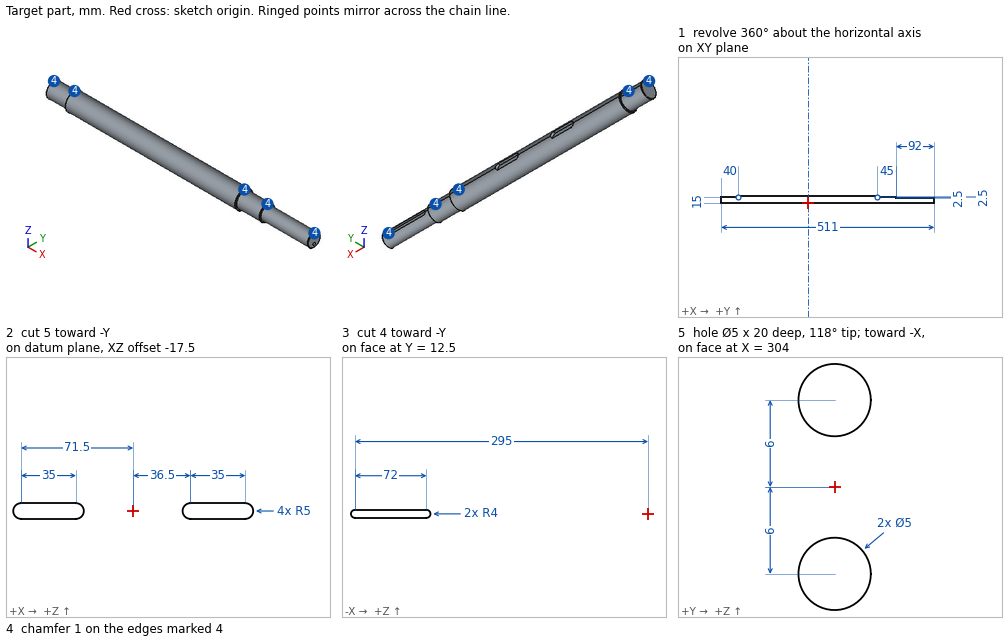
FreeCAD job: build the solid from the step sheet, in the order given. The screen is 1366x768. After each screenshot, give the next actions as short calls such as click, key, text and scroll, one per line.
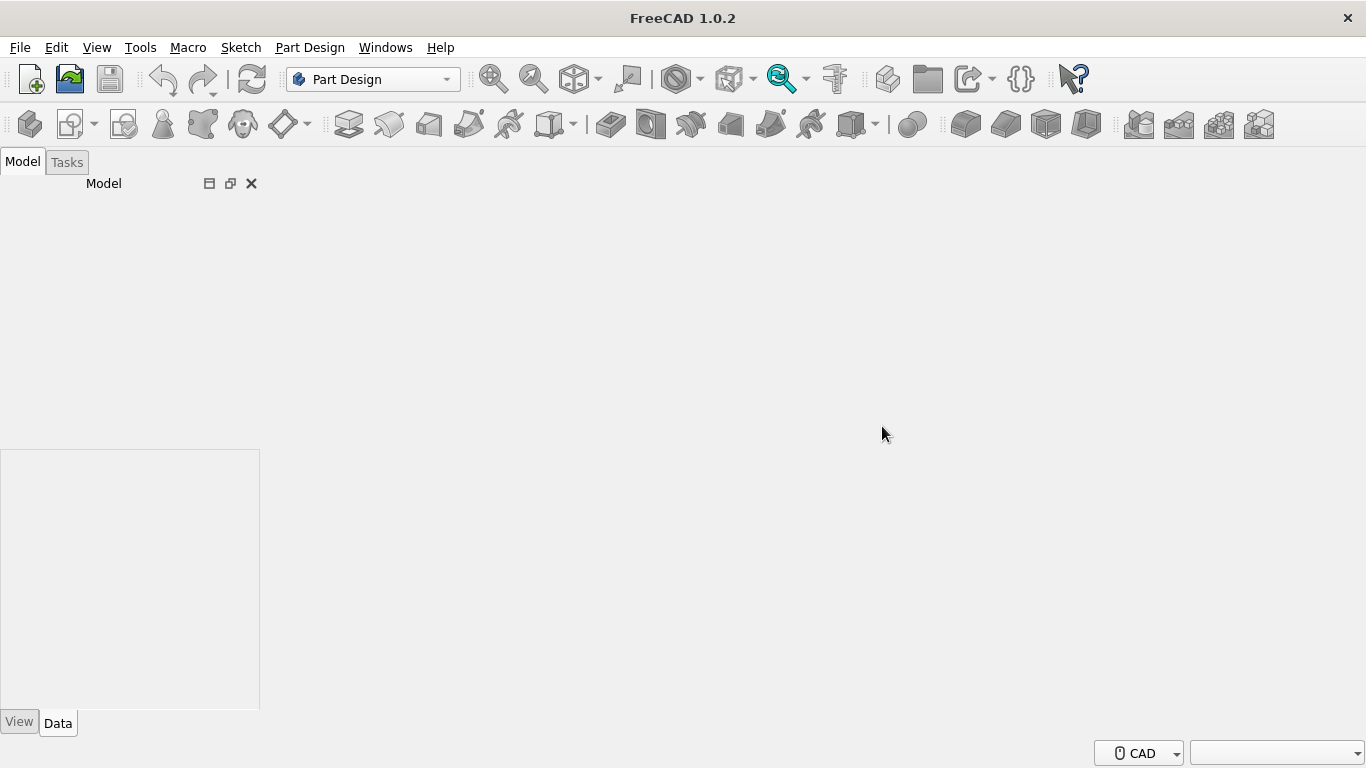
click(30, 80)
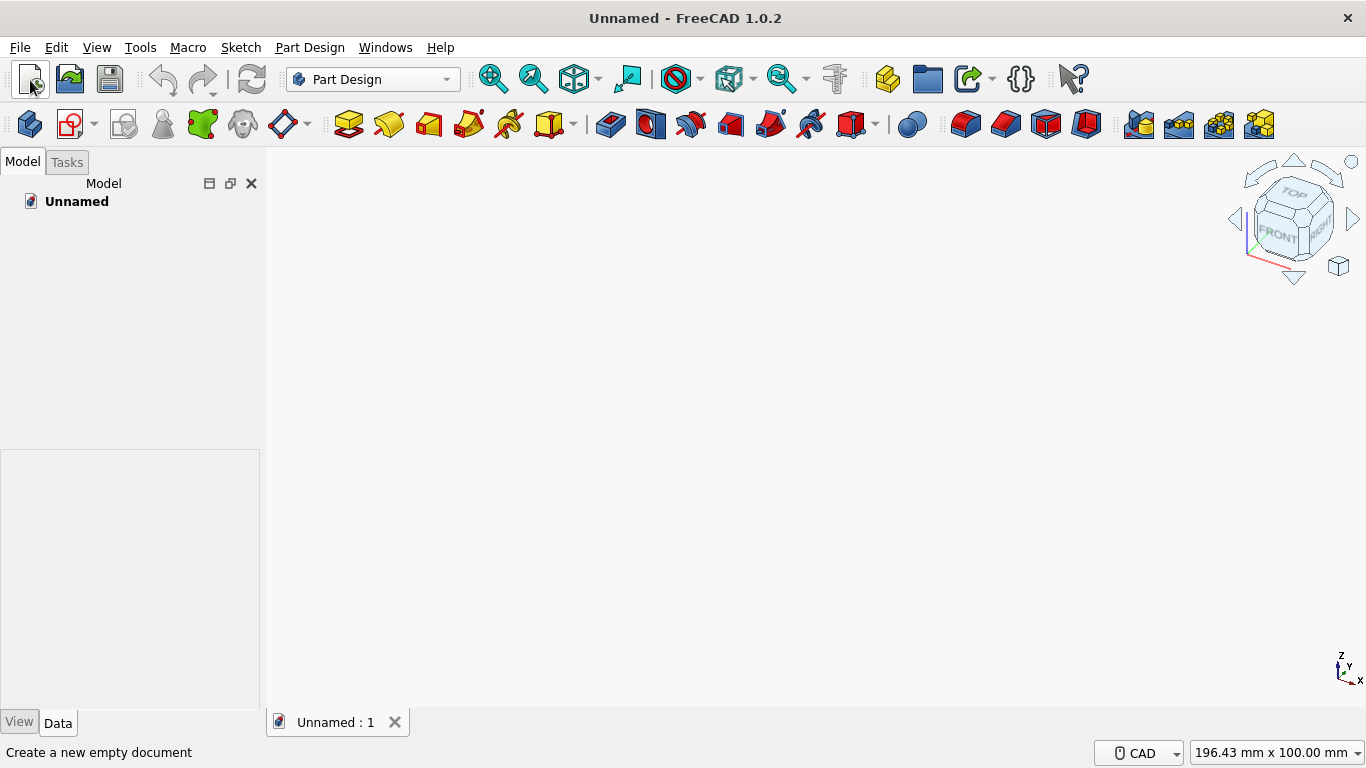
click(70, 124)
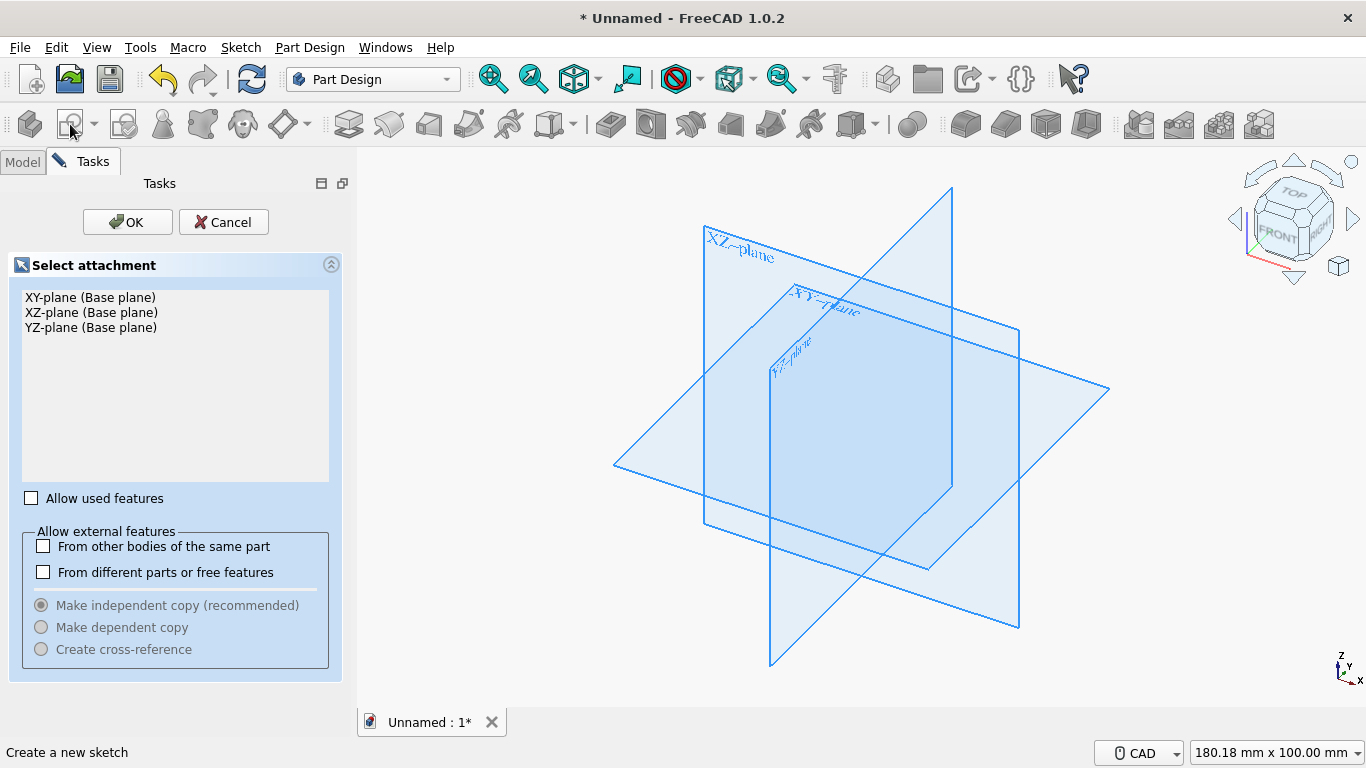
click(82, 298)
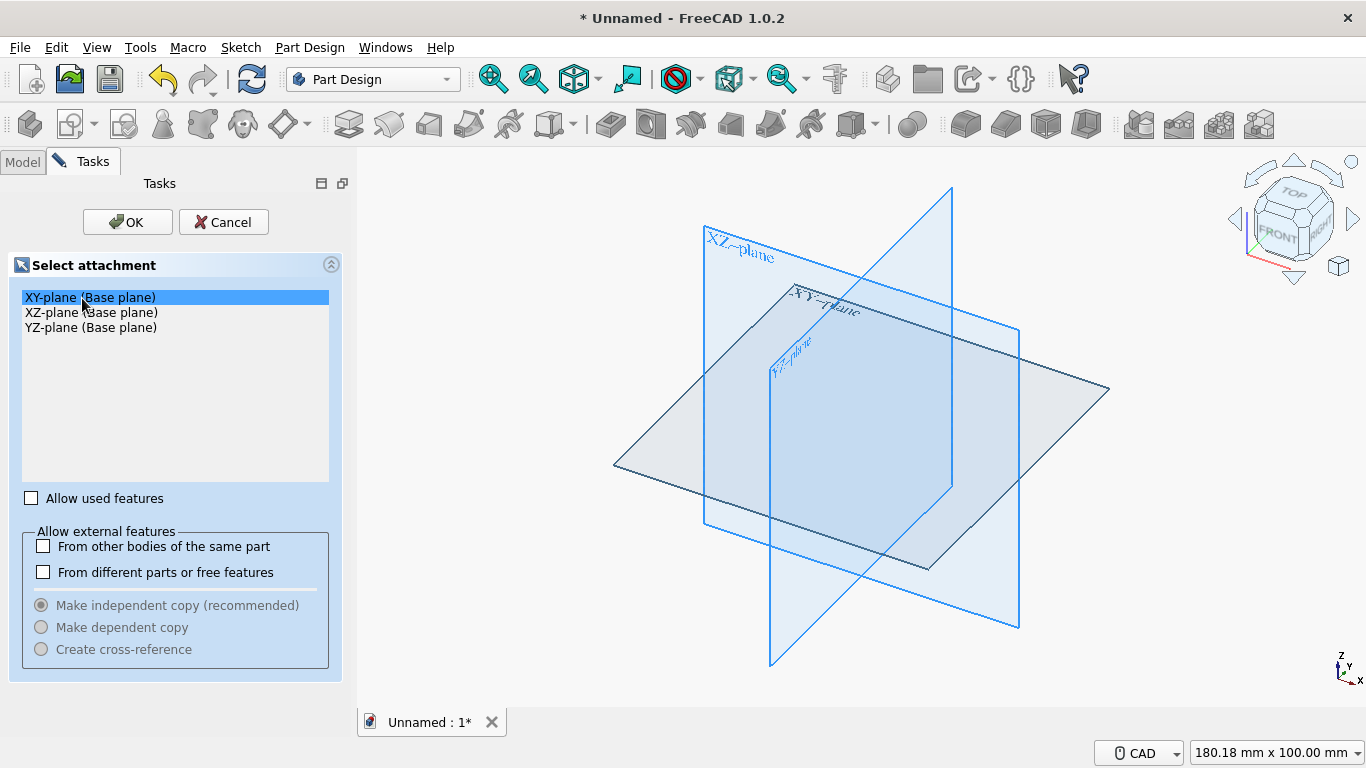
click(128, 222)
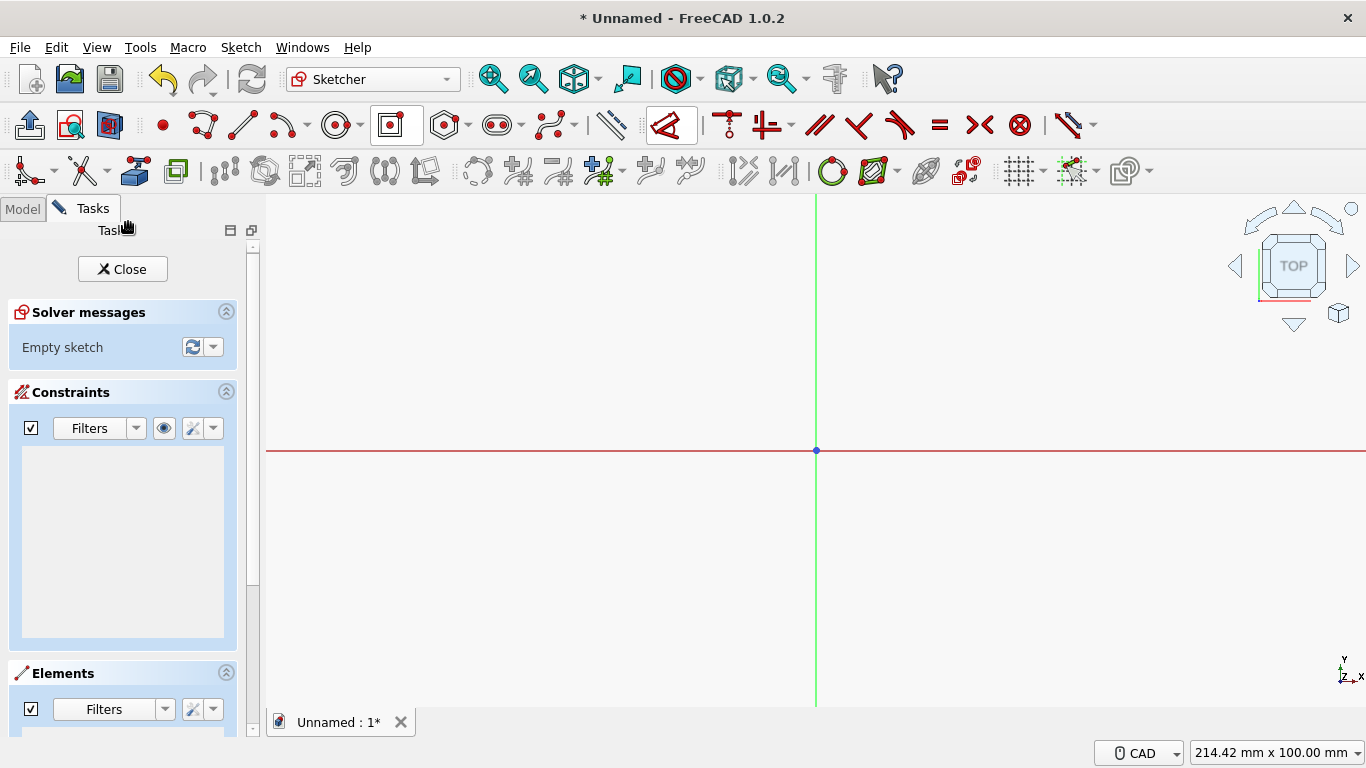
scroll(644, 465, down, 7)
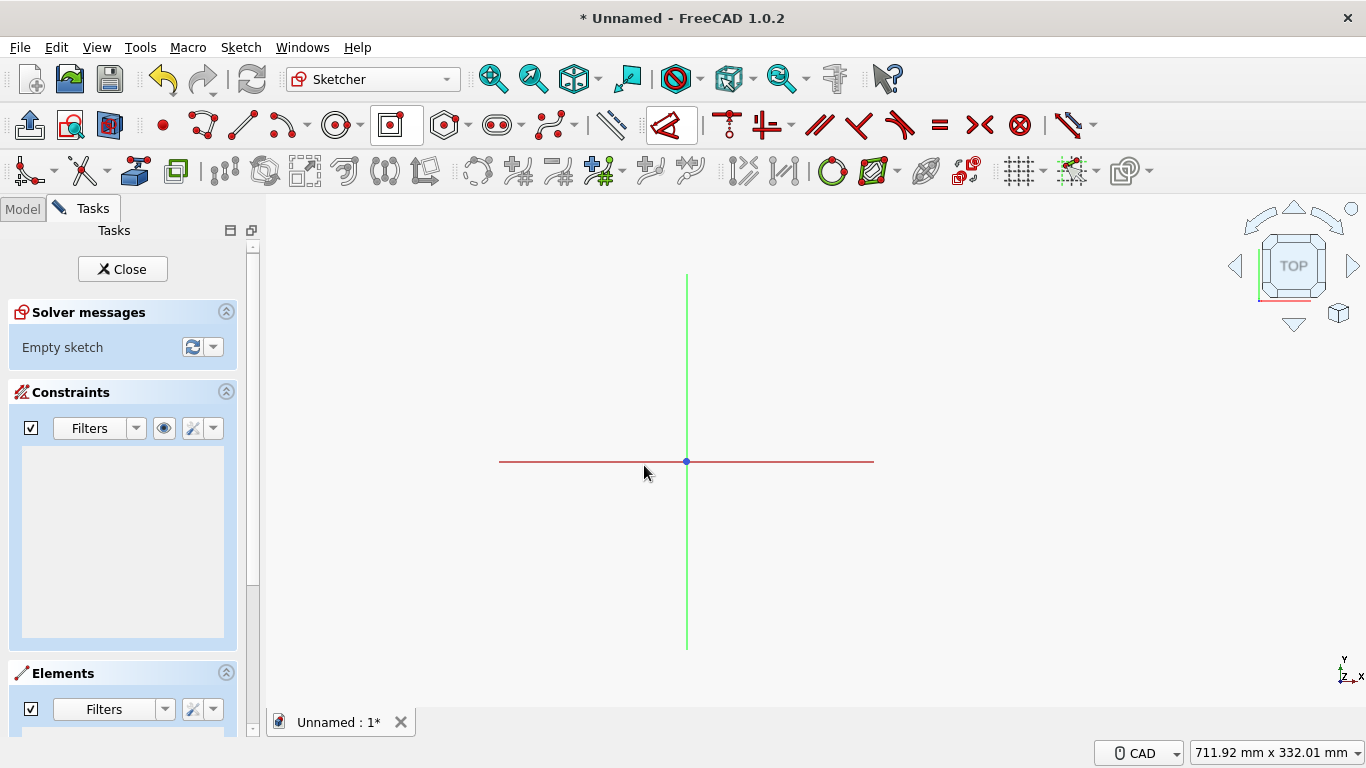
click(204, 126)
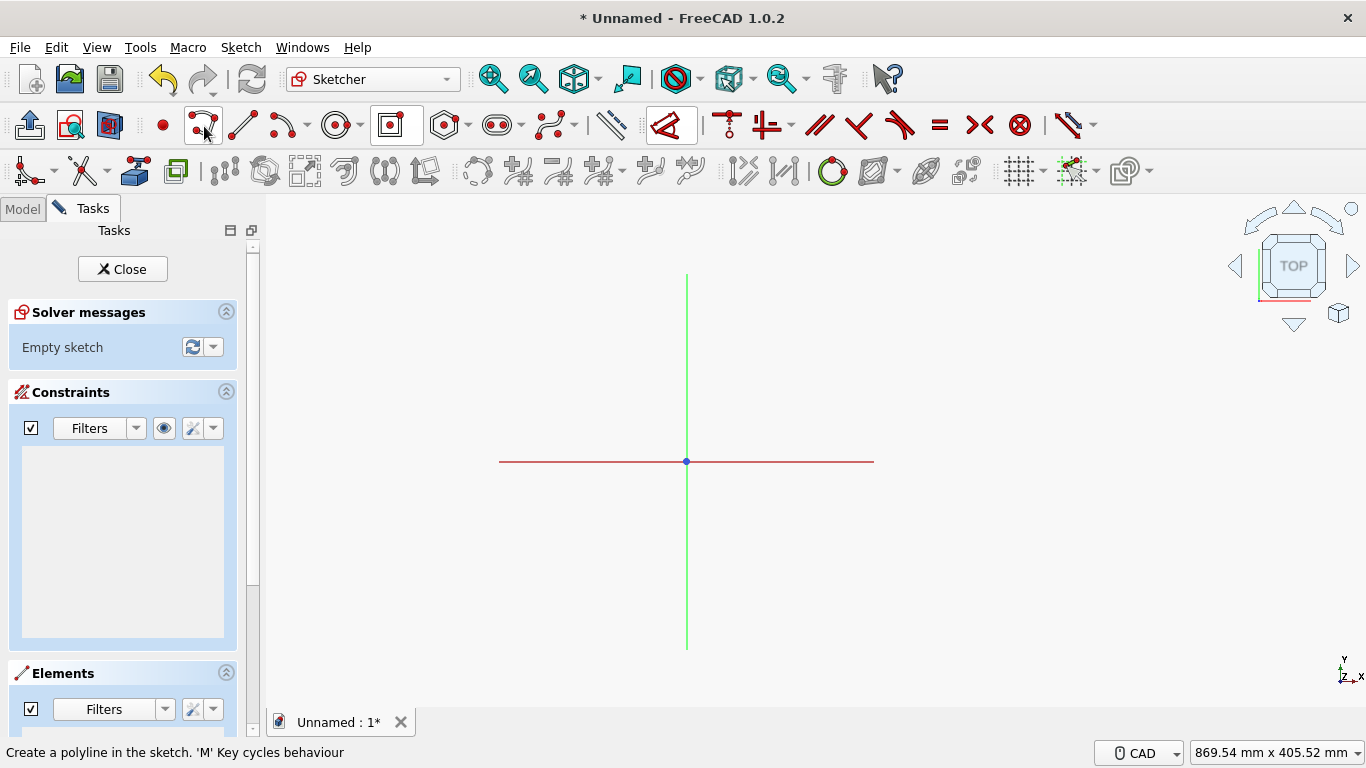
click(475, 443)
click(425, 443)
click(425, 462)
click(1071, 453)
click(1071, 446)
click(955, 446)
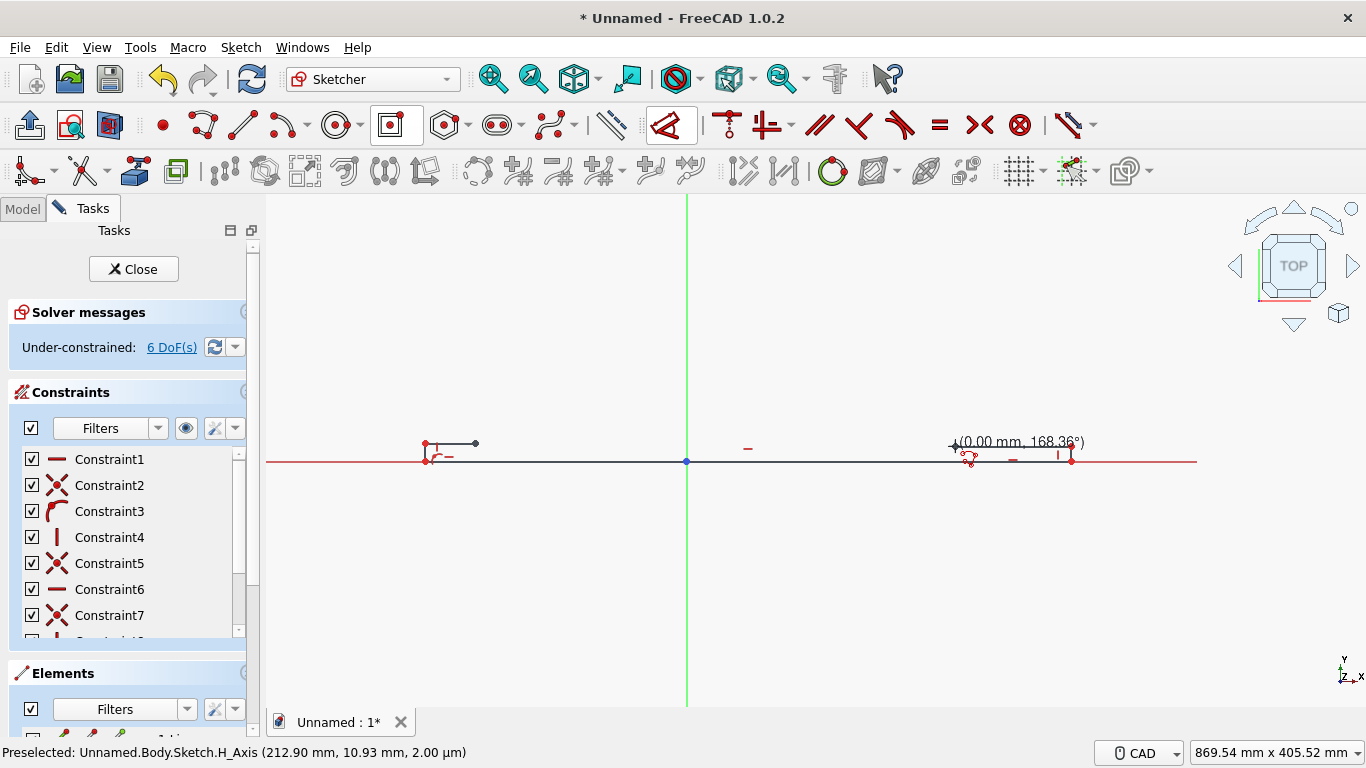
scroll(955, 443, up, 9)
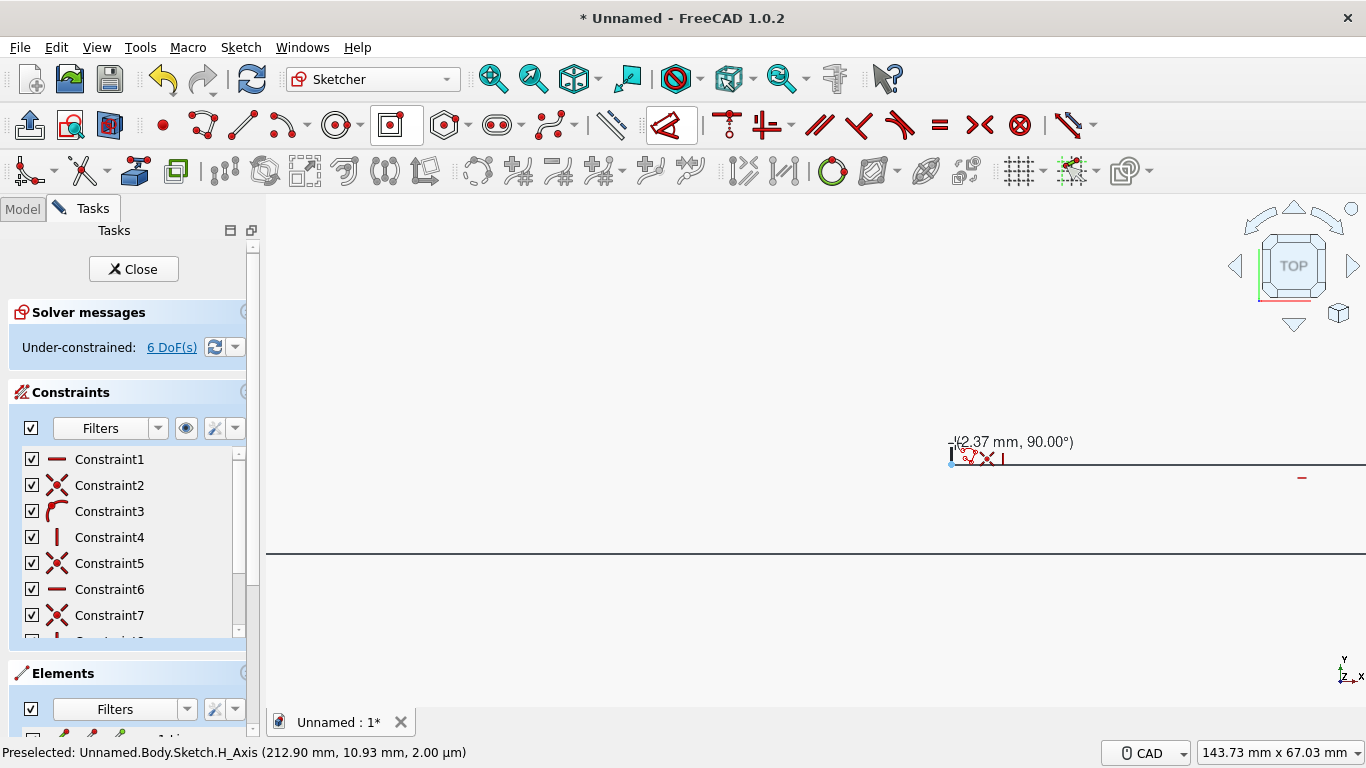
click(952, 440)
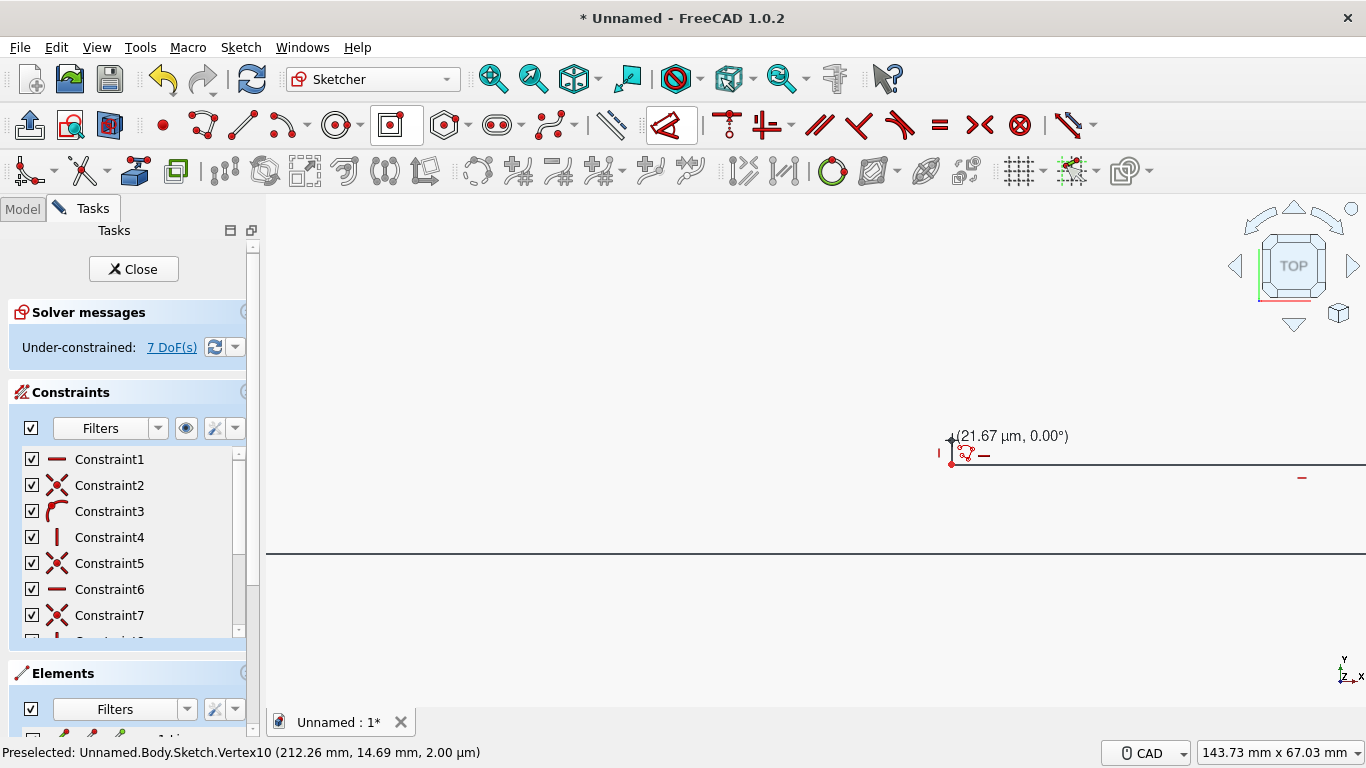
scroll(955, 443, down, 9)